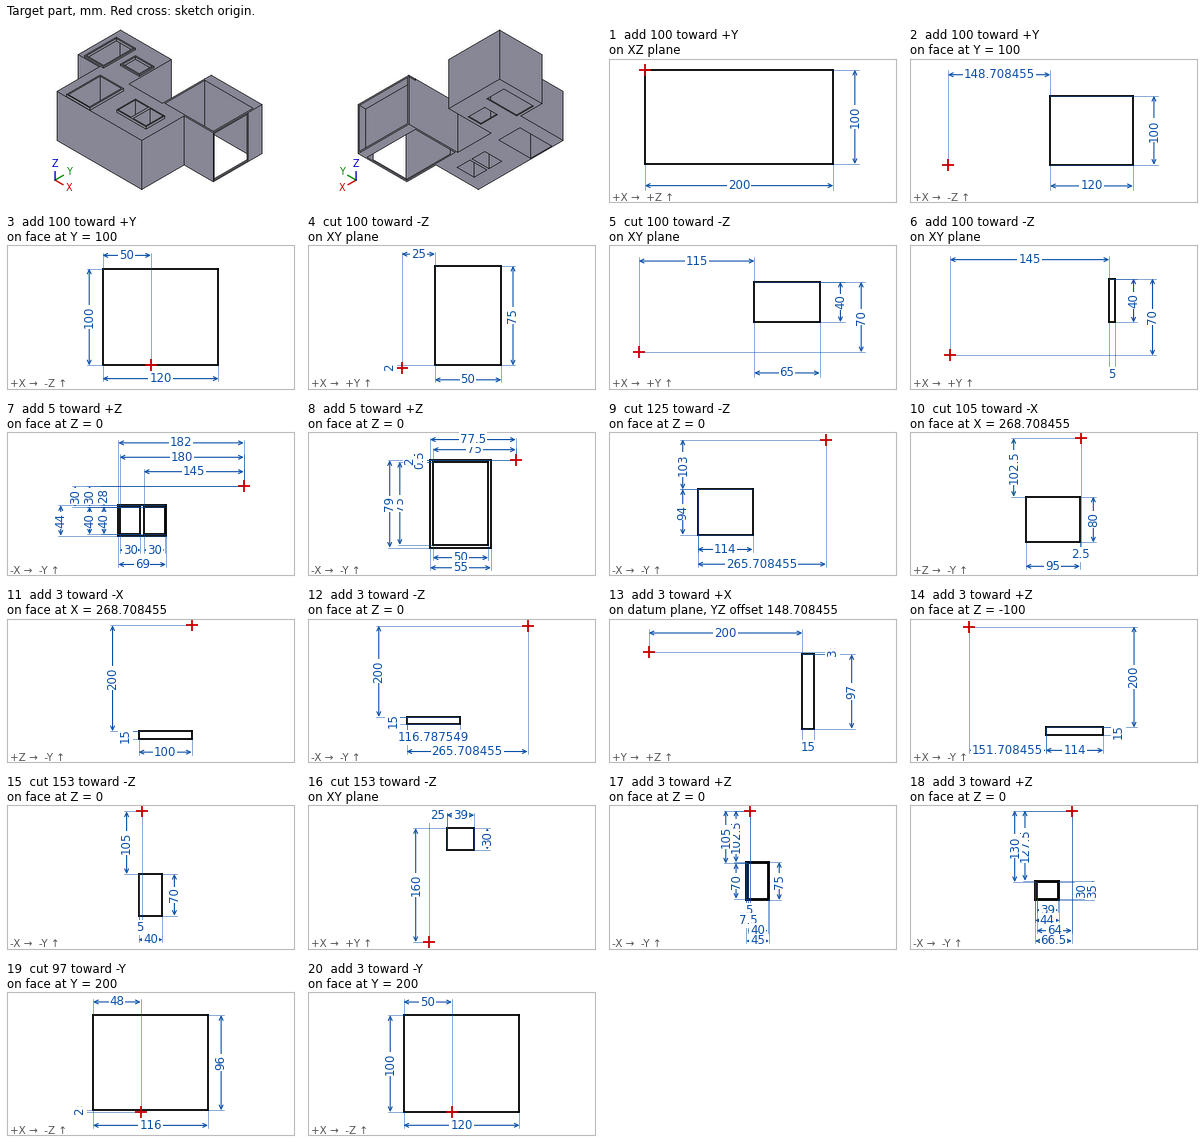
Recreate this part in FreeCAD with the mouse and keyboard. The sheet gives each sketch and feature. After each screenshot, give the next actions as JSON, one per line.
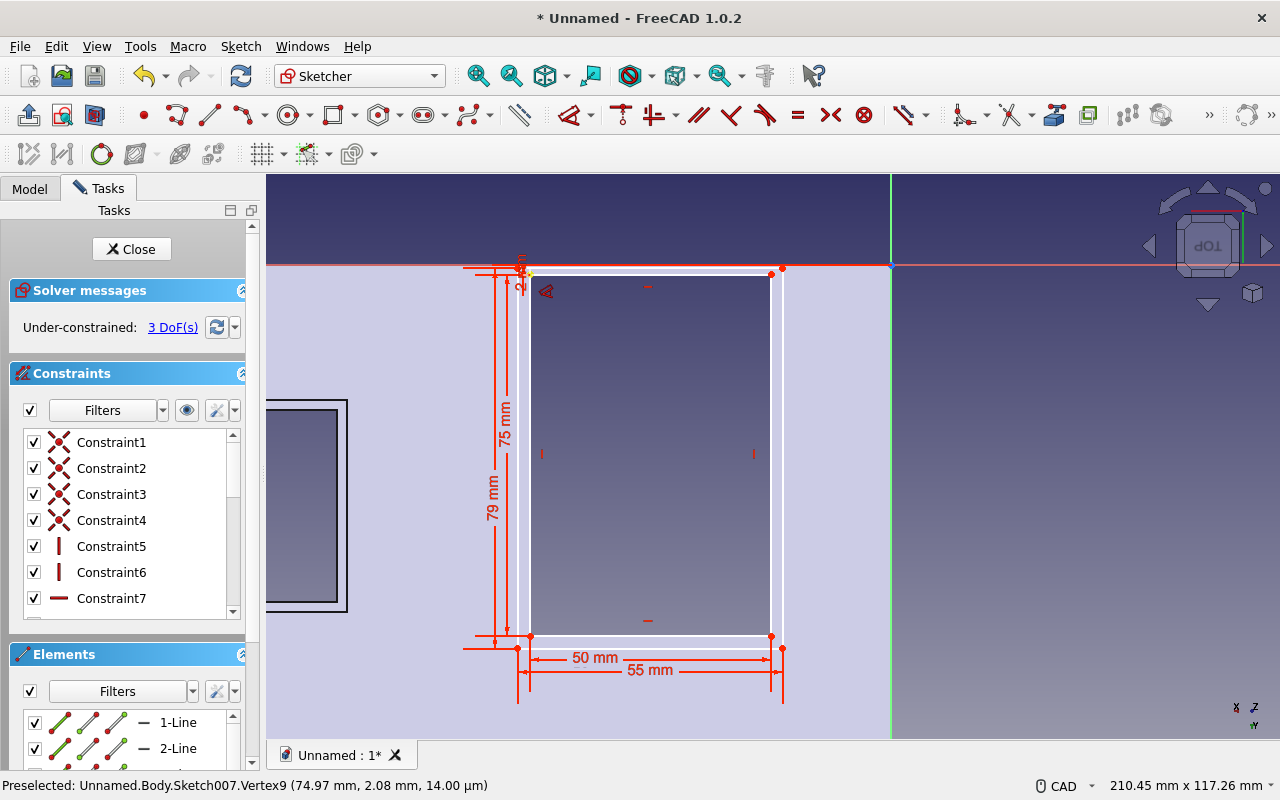
{"action": "left_click", "coordinate": [530, 275]}
{"action": "left_click", "coordinate": [711, 231]}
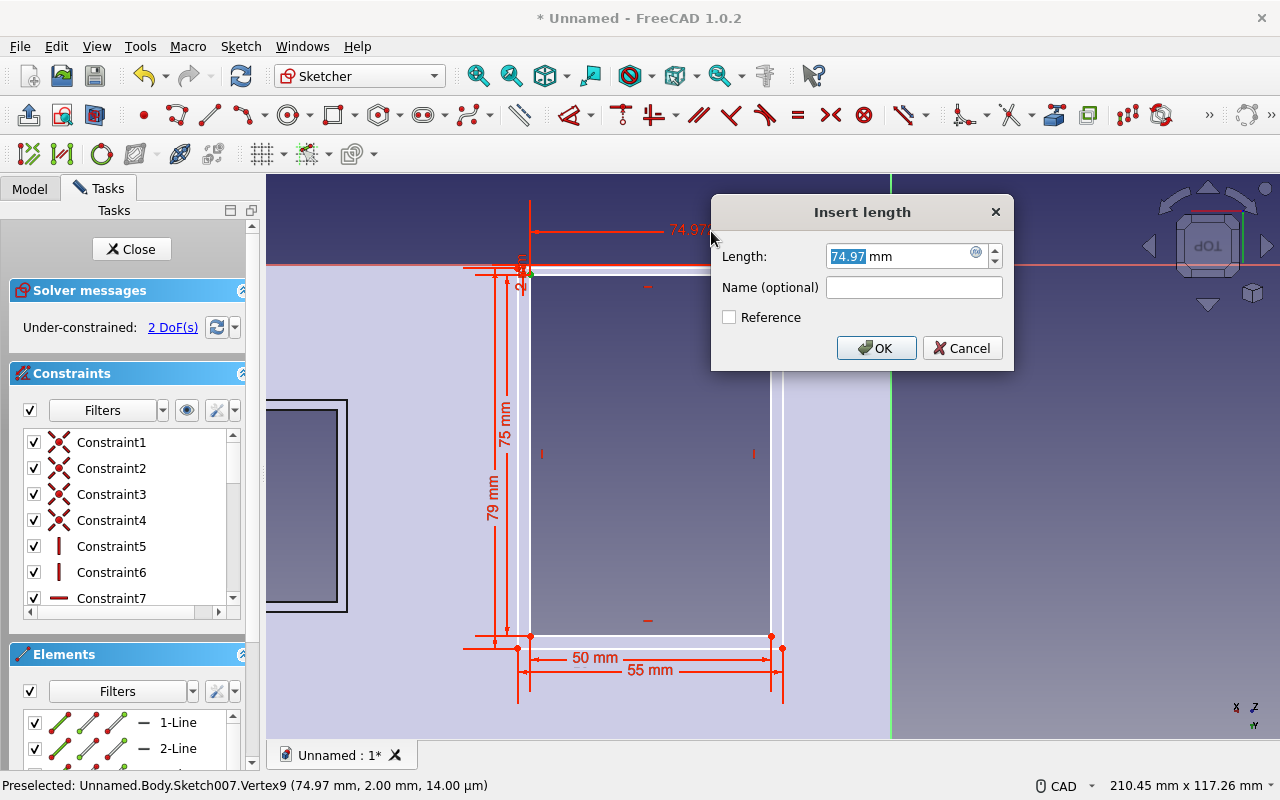
{"action": "type", "text": "75"}
{"action": "key", "text": "Return"}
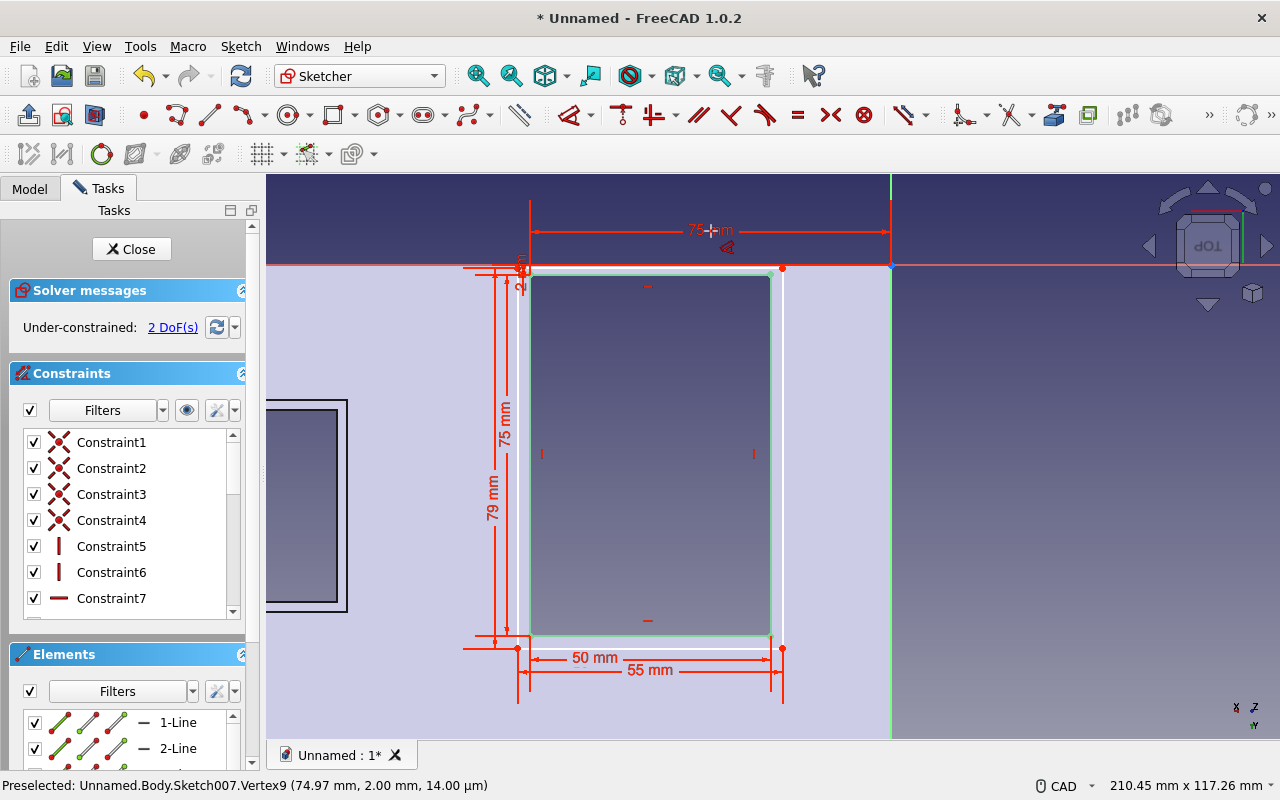
{"action": "scroll", "coordinate": [518, 268], "scroll_direction": "up", "scroll_amount": 15}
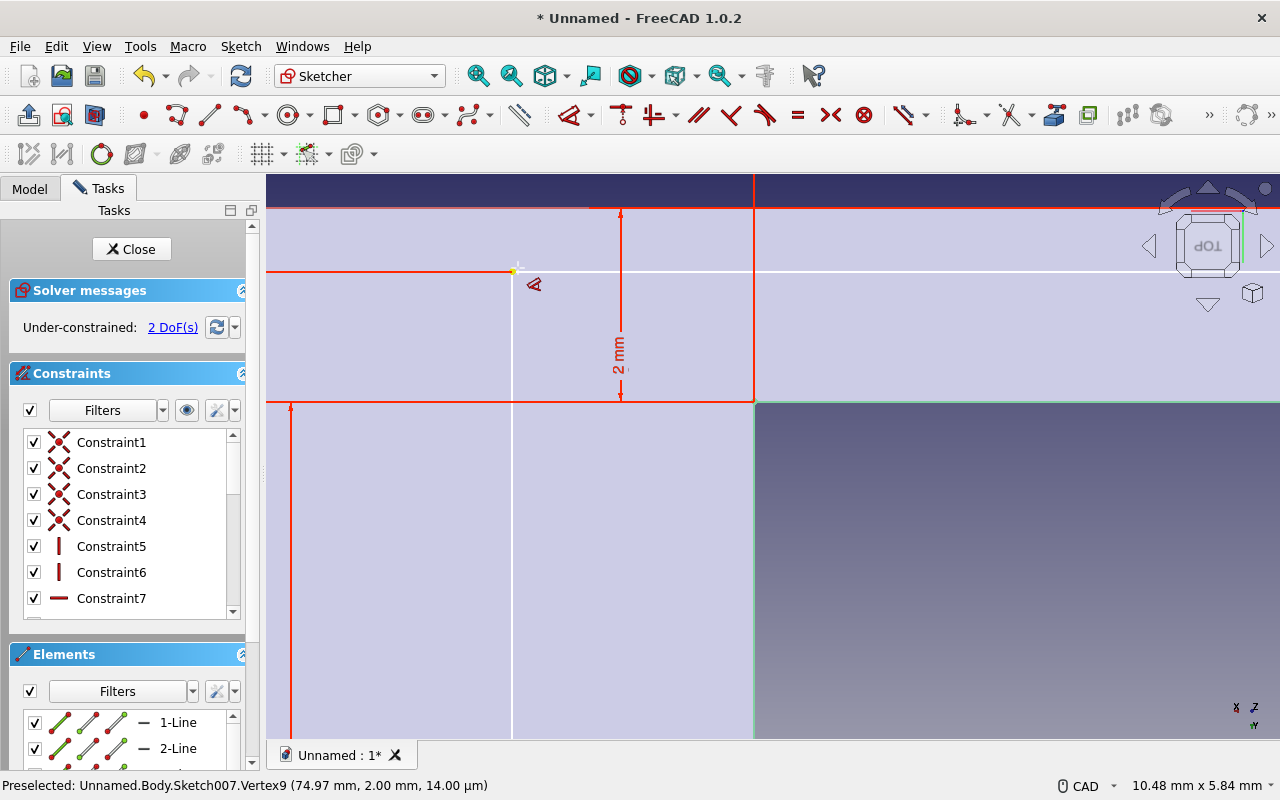
{"action": "left_click", "coordinate": [512, 272]}
{"action": "left_click", "coordinate": [478, 240]}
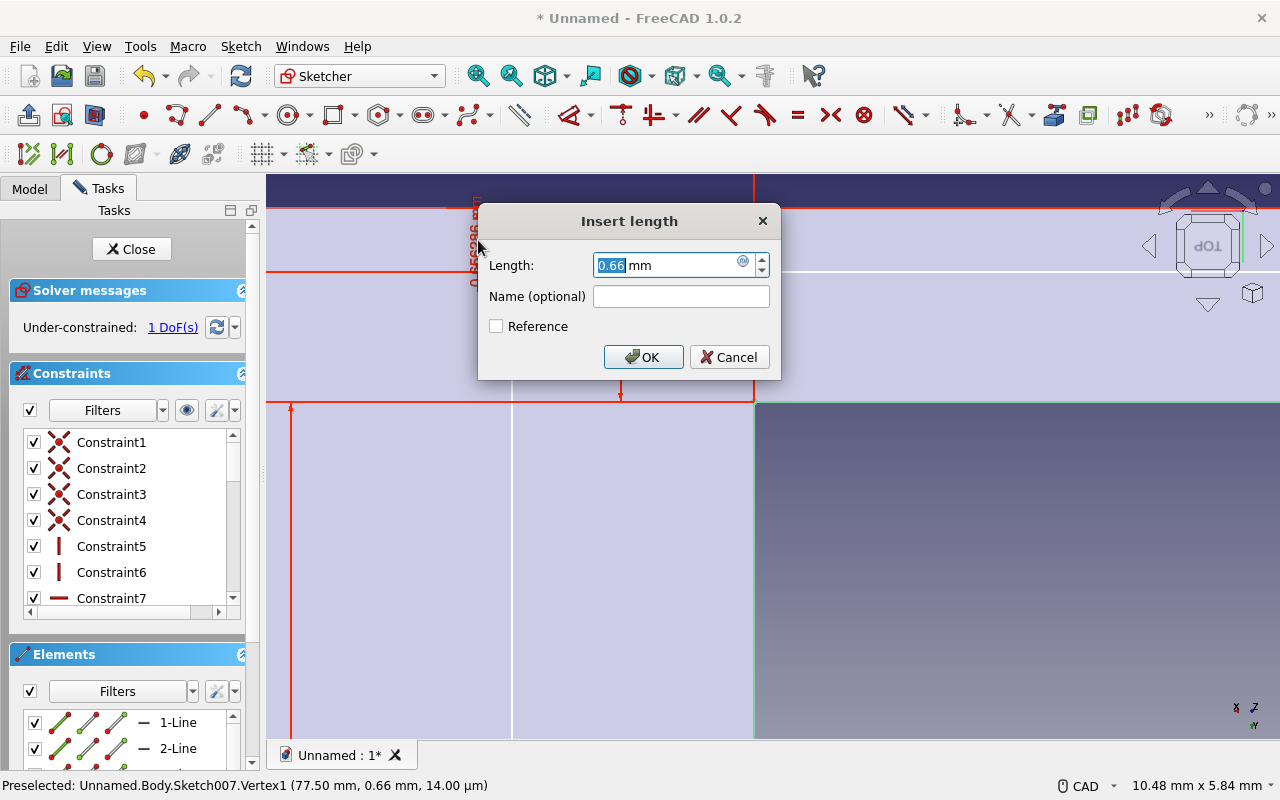
{"action": "type", "text": "0.5"}
{"action": "key", "text": "Return"}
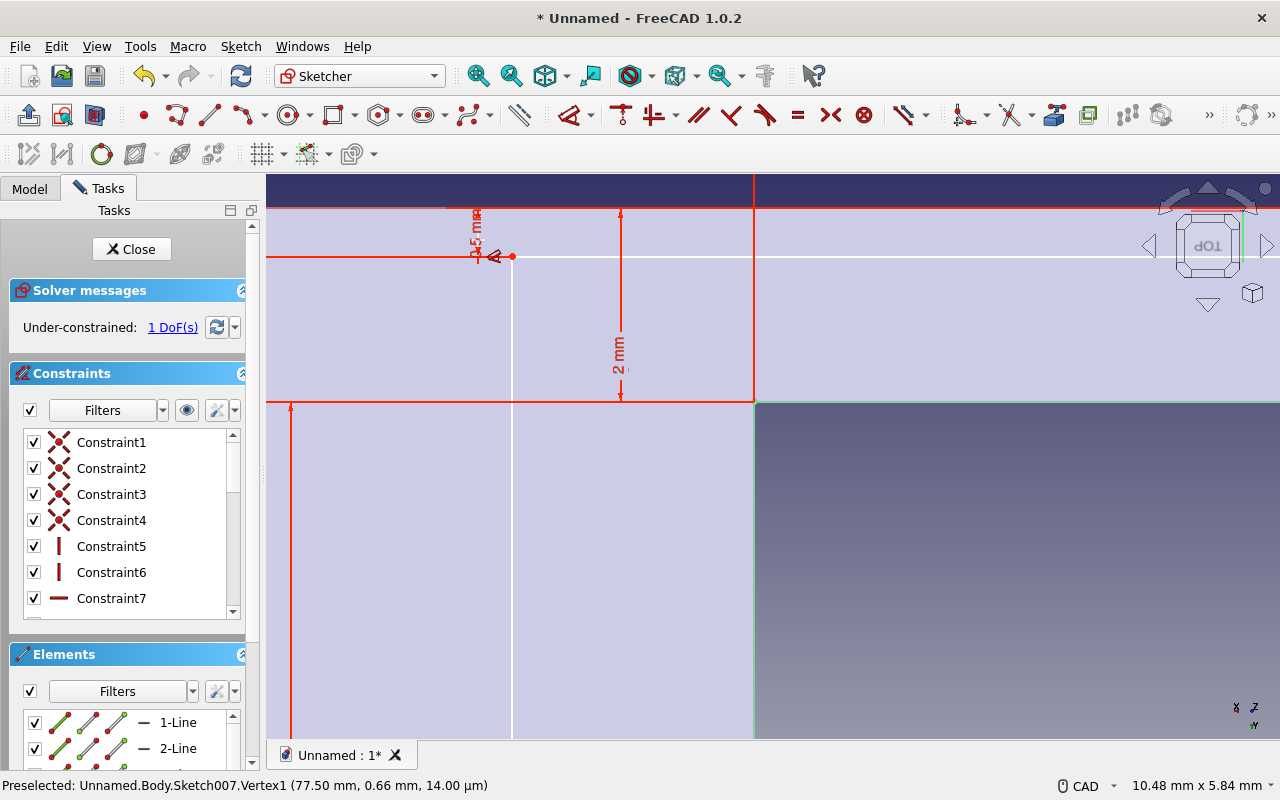
{"action": "scroll", "coordinate": [518, 268], "scroll_direction": "down", "scroll_amount": 15}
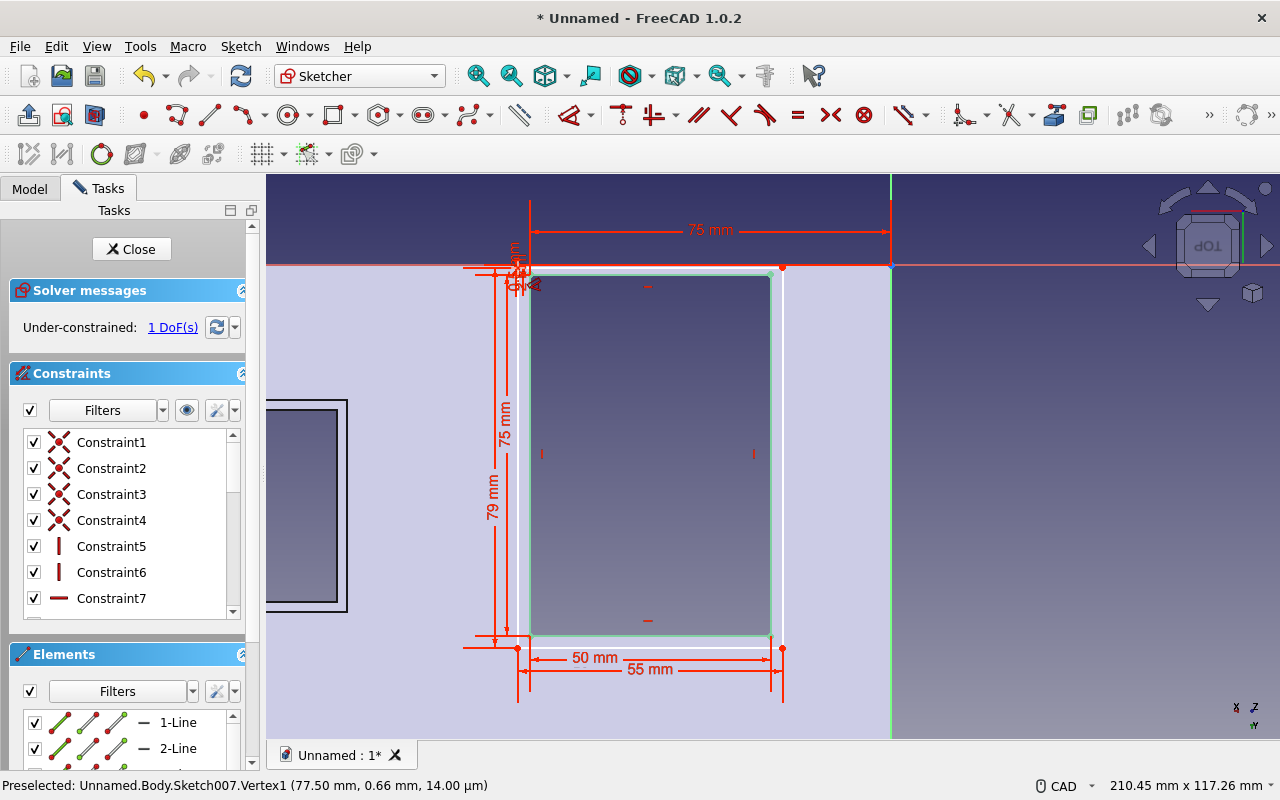
{"action": "left_click", "coordinate": [518, 268]}
{"action": "left_click", "coordinate": [619, 231]}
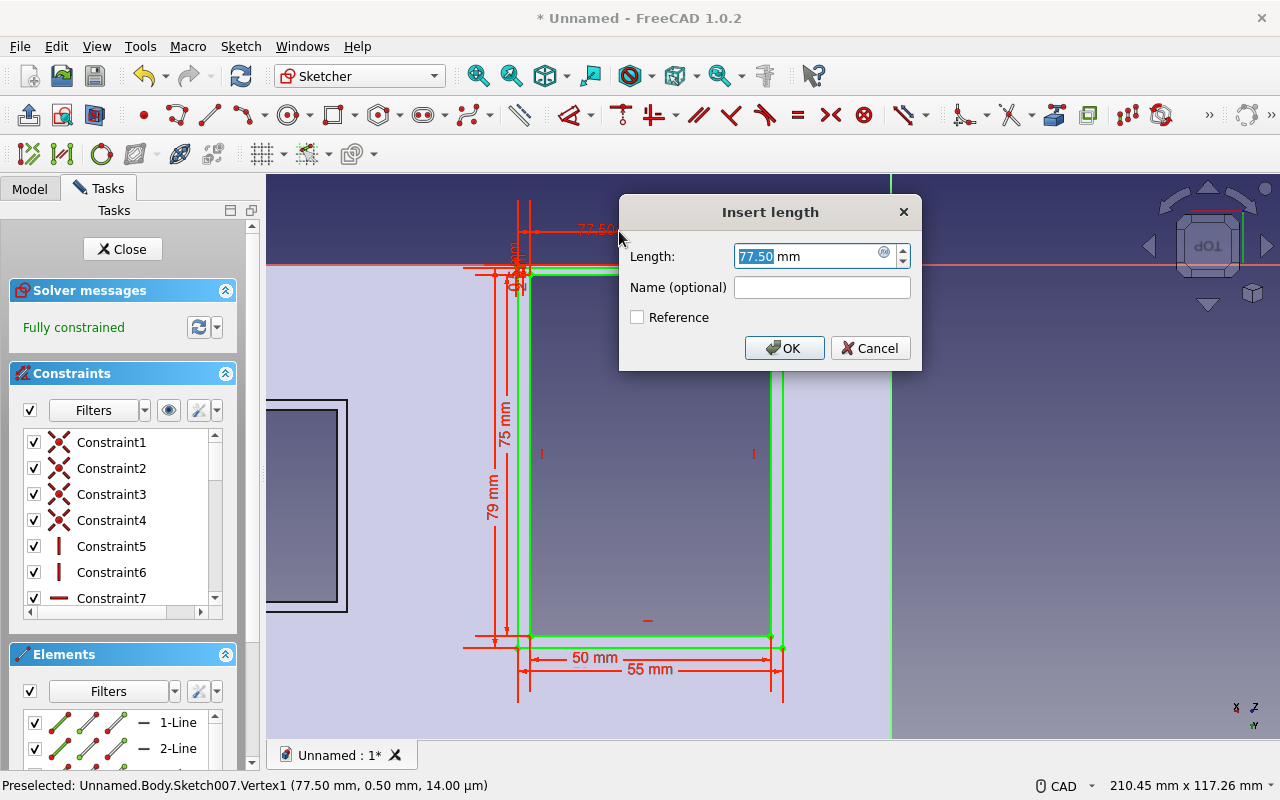
{"action": "type", "text": "77.5"}
{"action": "key", "text": "Return"}
{"action": "key", "text": "Escape"}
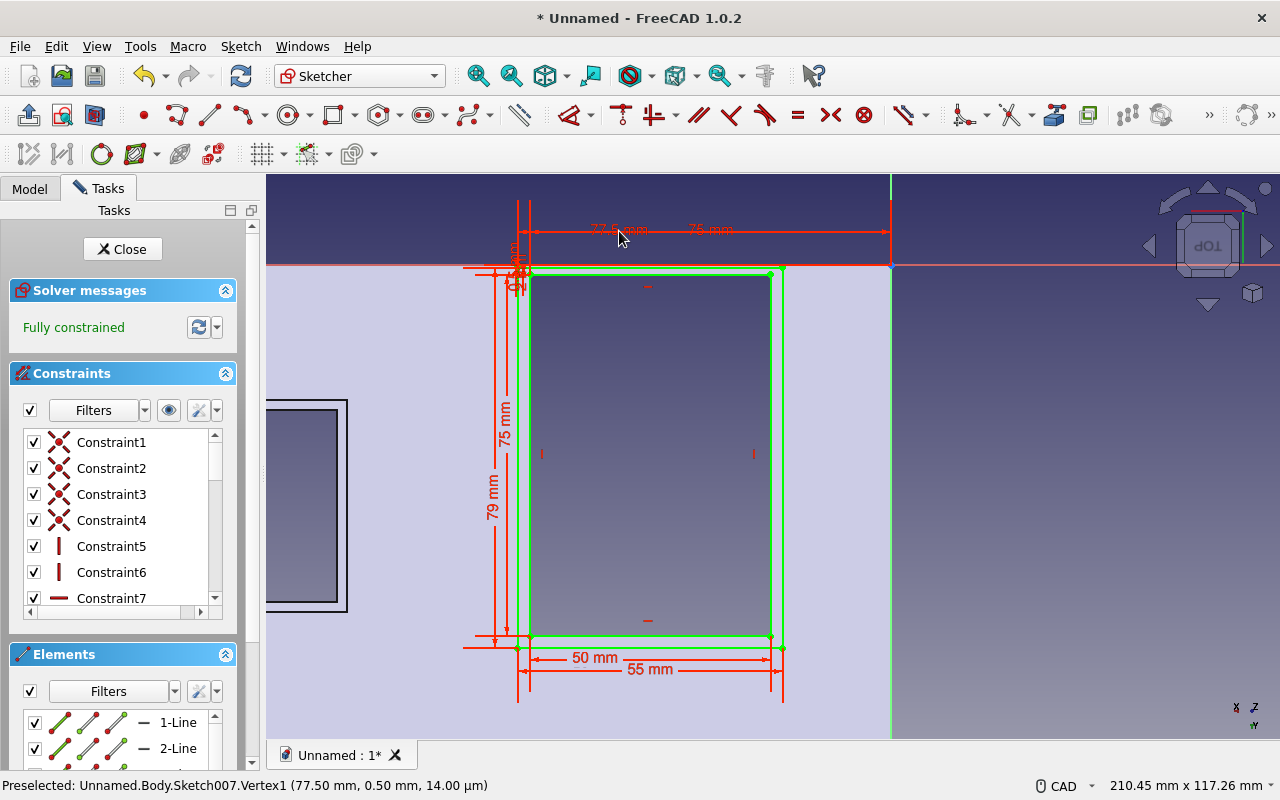
{"action": "left_click", "coordinate": [123, 249]}